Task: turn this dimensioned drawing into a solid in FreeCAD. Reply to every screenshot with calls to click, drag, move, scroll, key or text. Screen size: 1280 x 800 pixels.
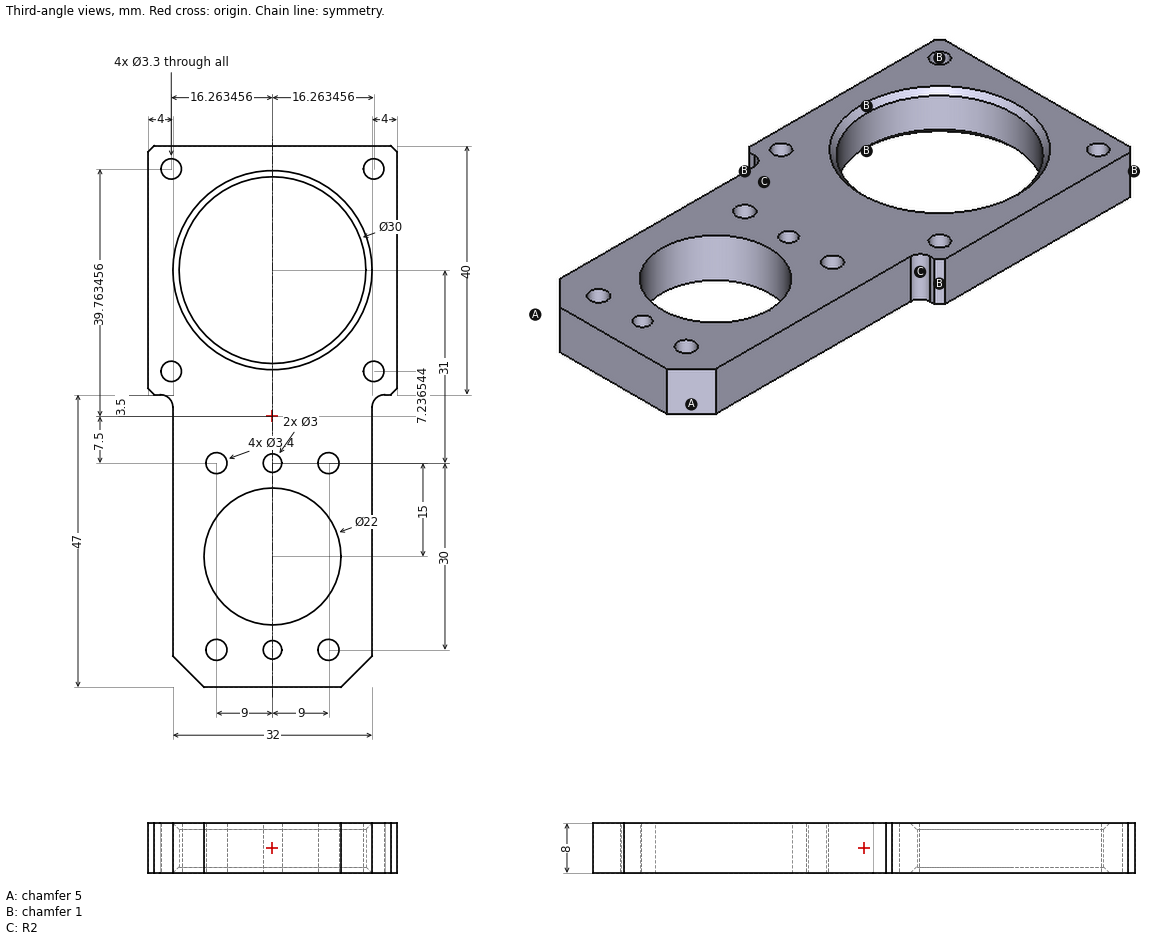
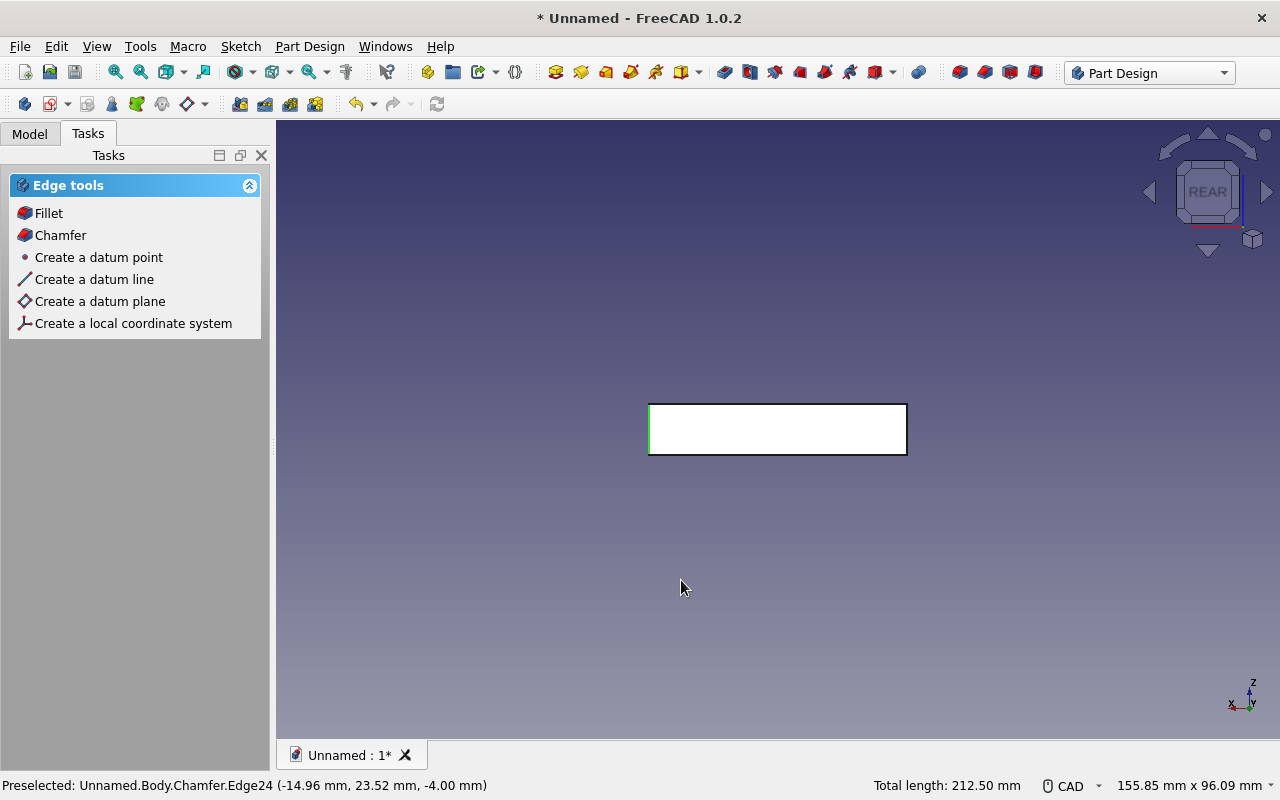
click(907, 429, ctrl)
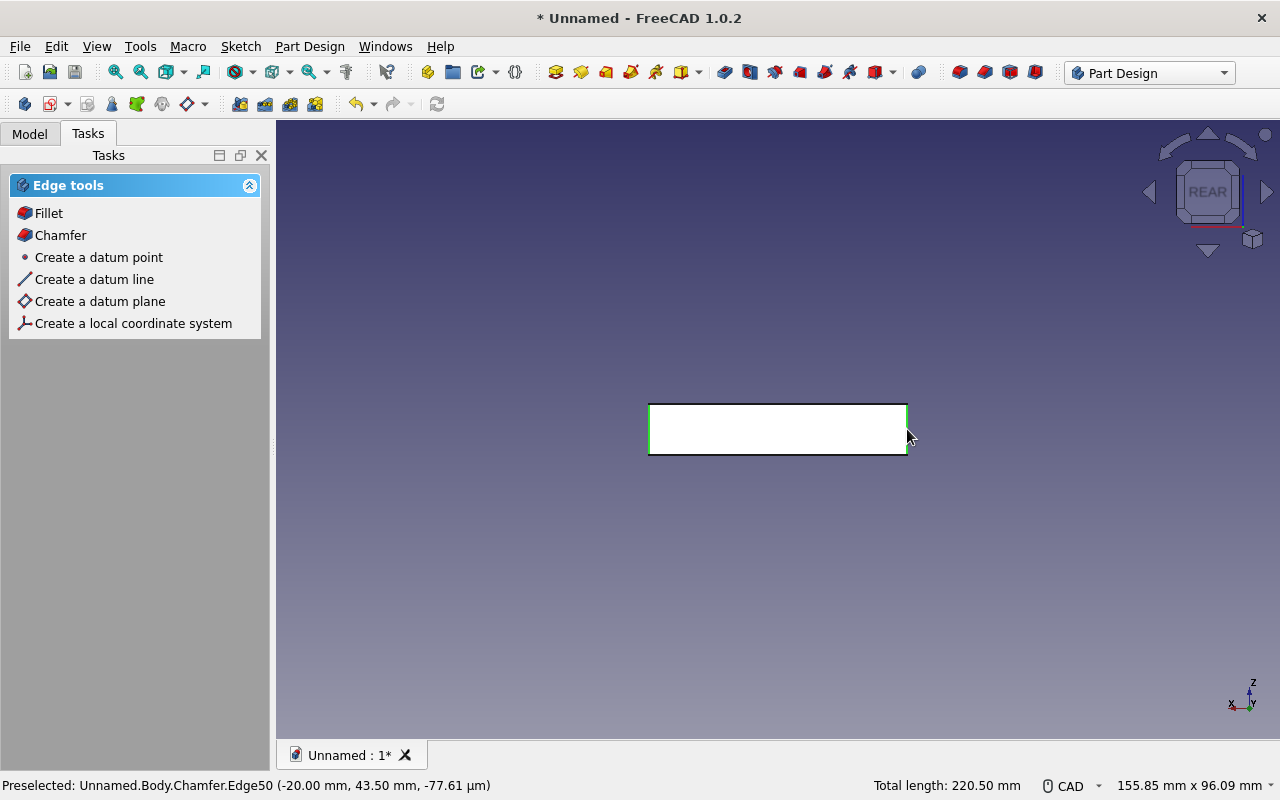
click(985, 72)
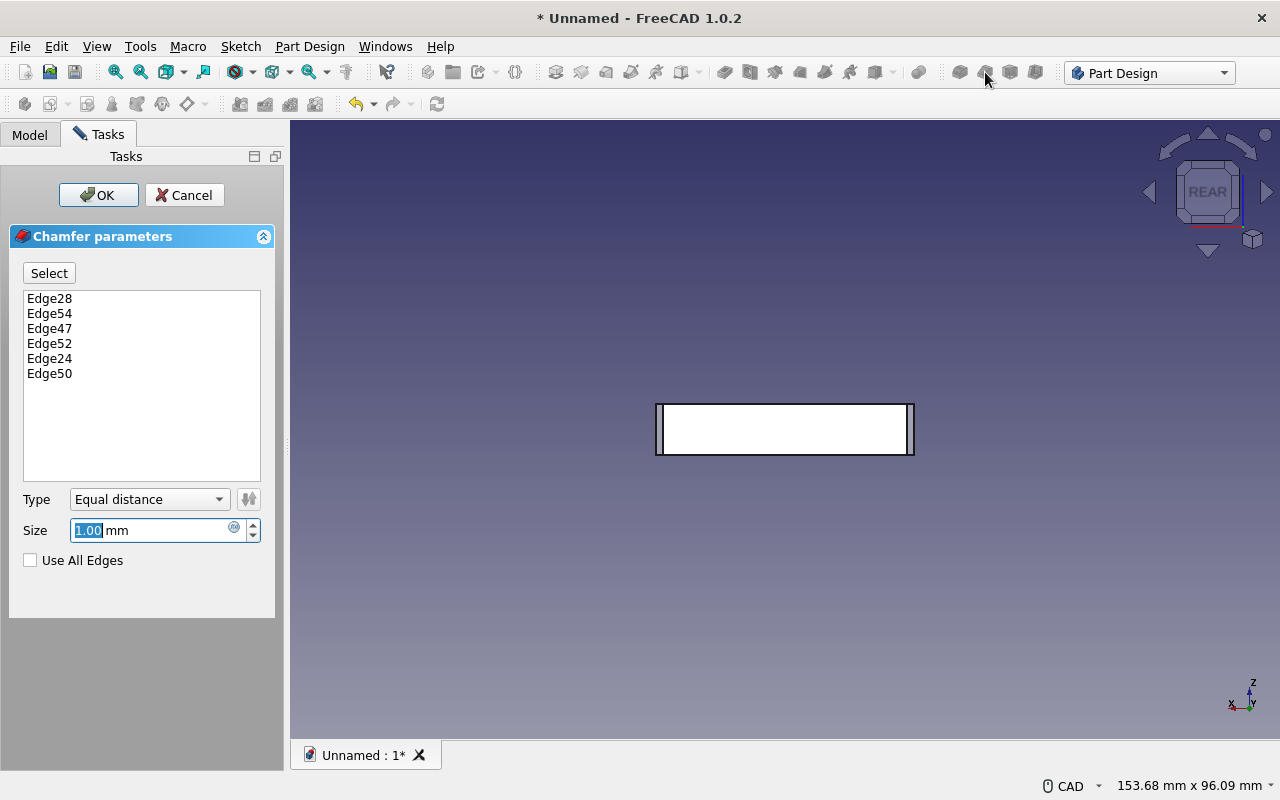
text(1)
key(Tab)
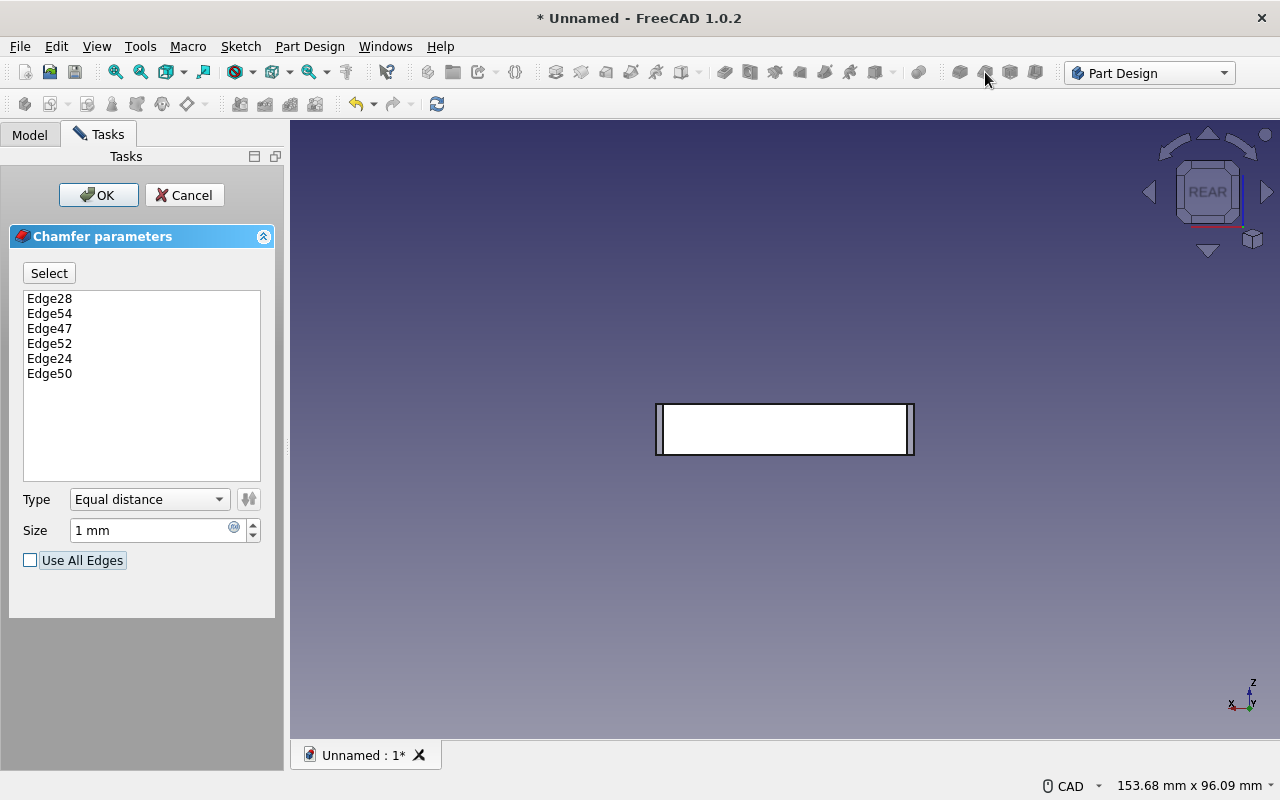
click(99, 195)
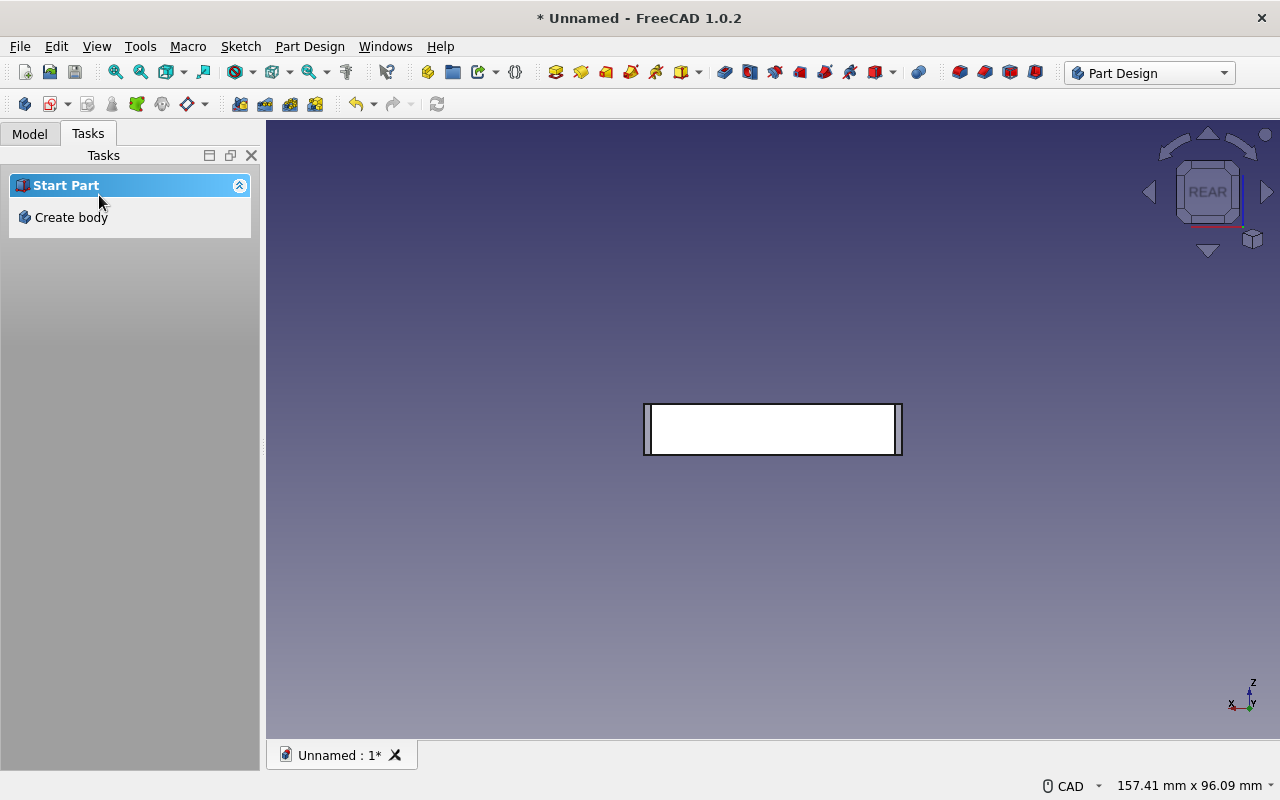
key(v)
key(f)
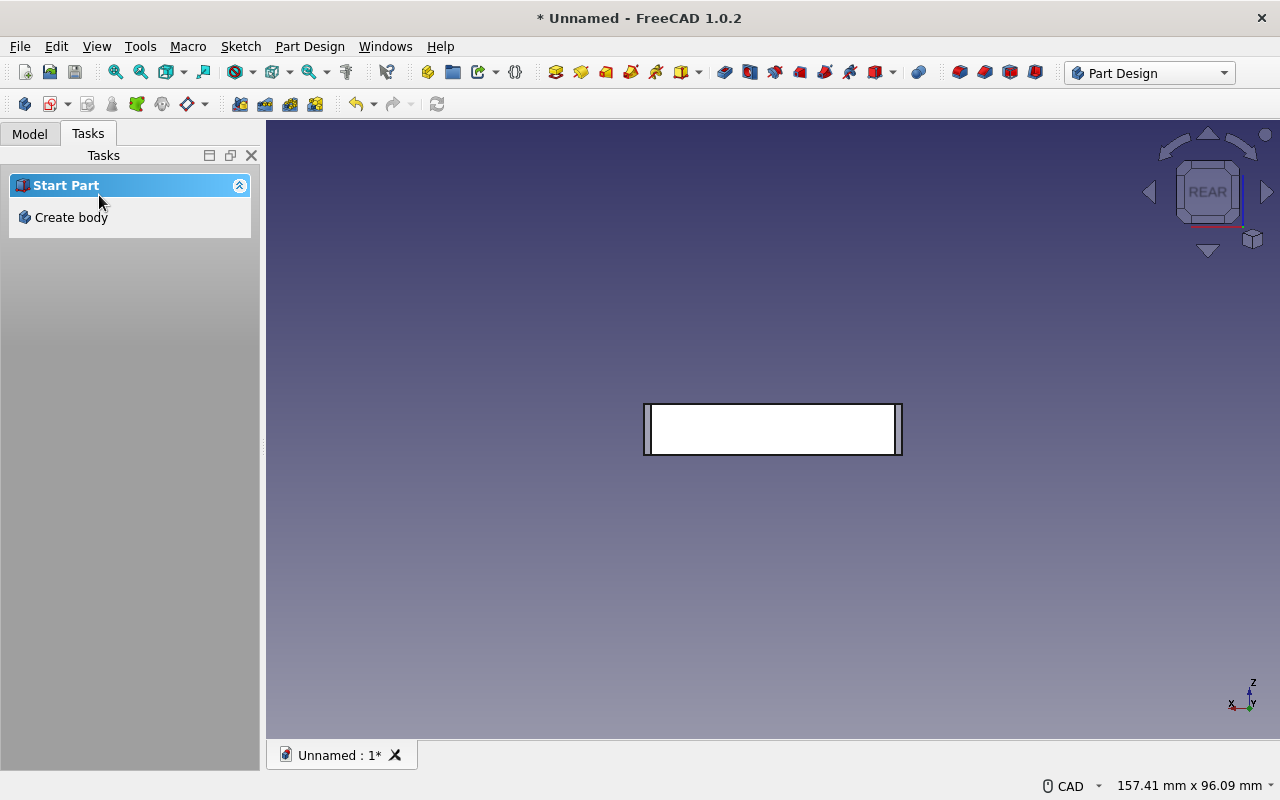
key(0)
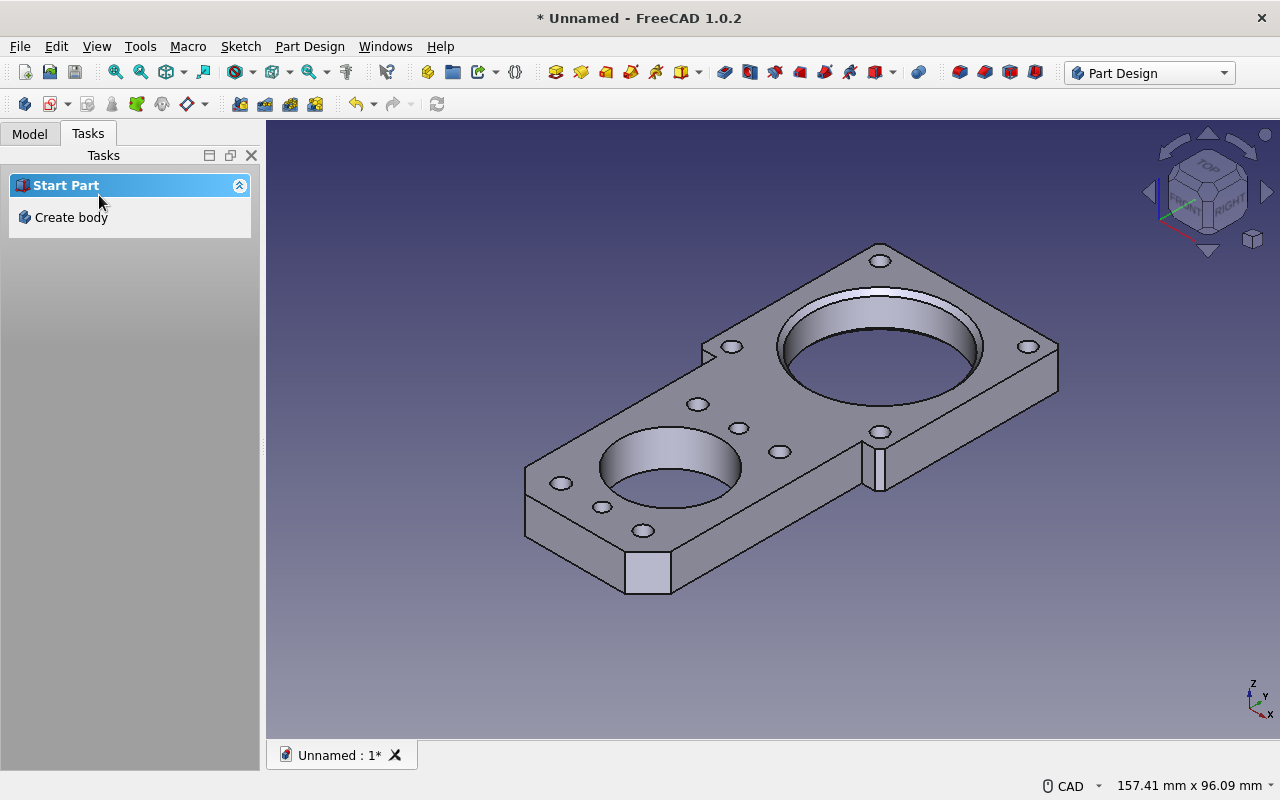
key(2)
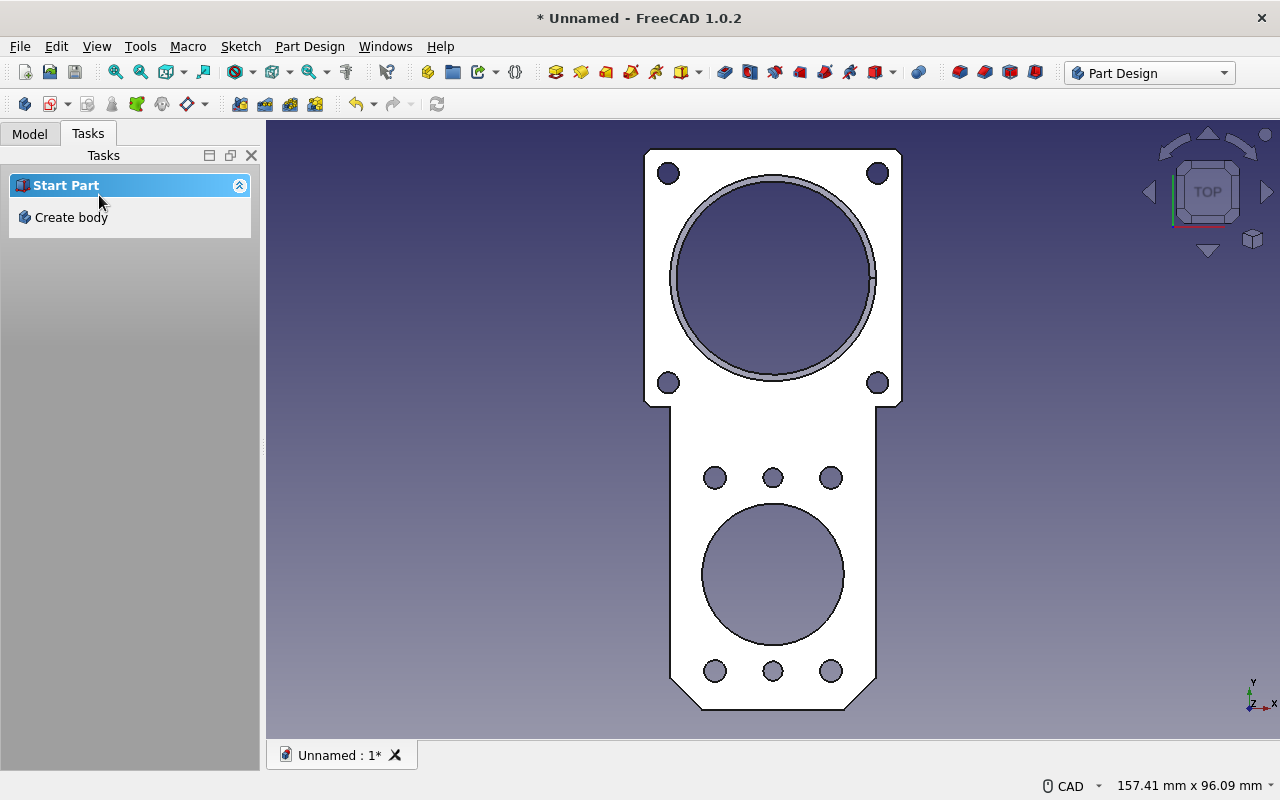
key(1)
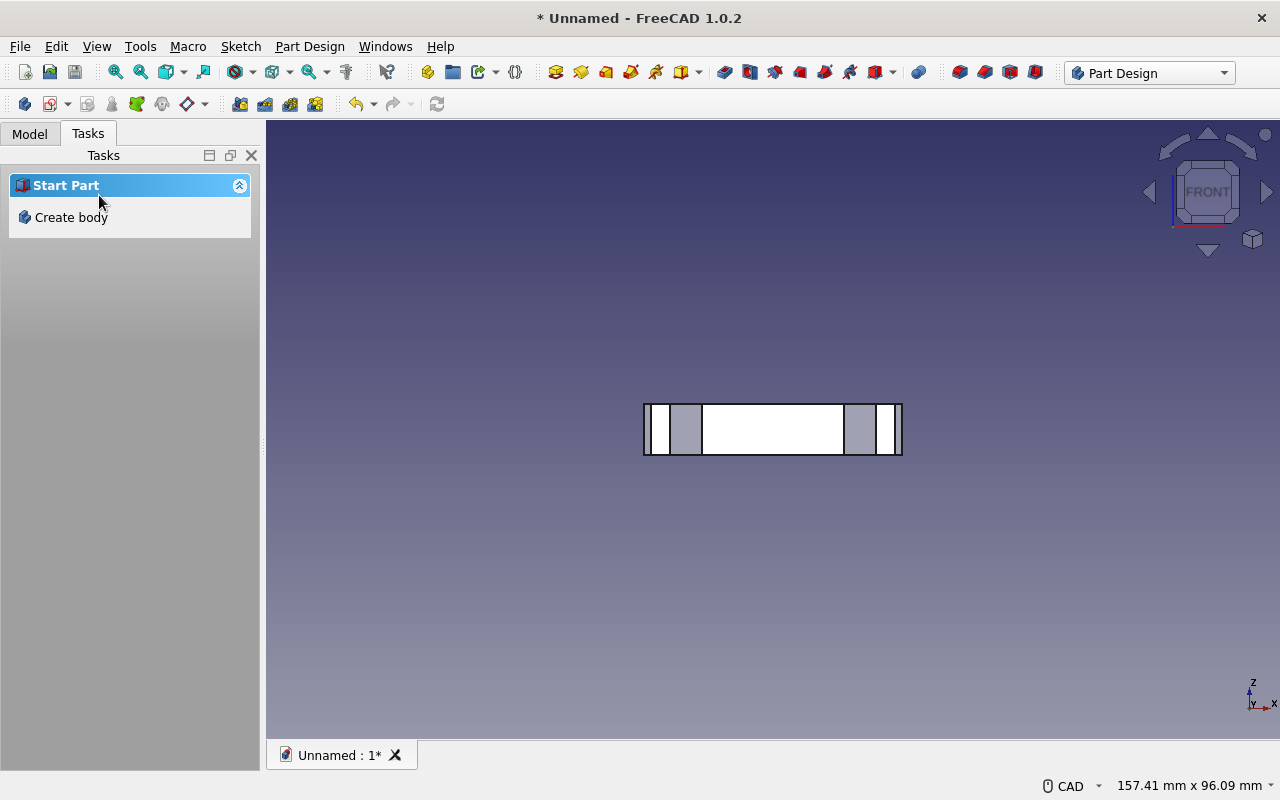
key(v)
key(f)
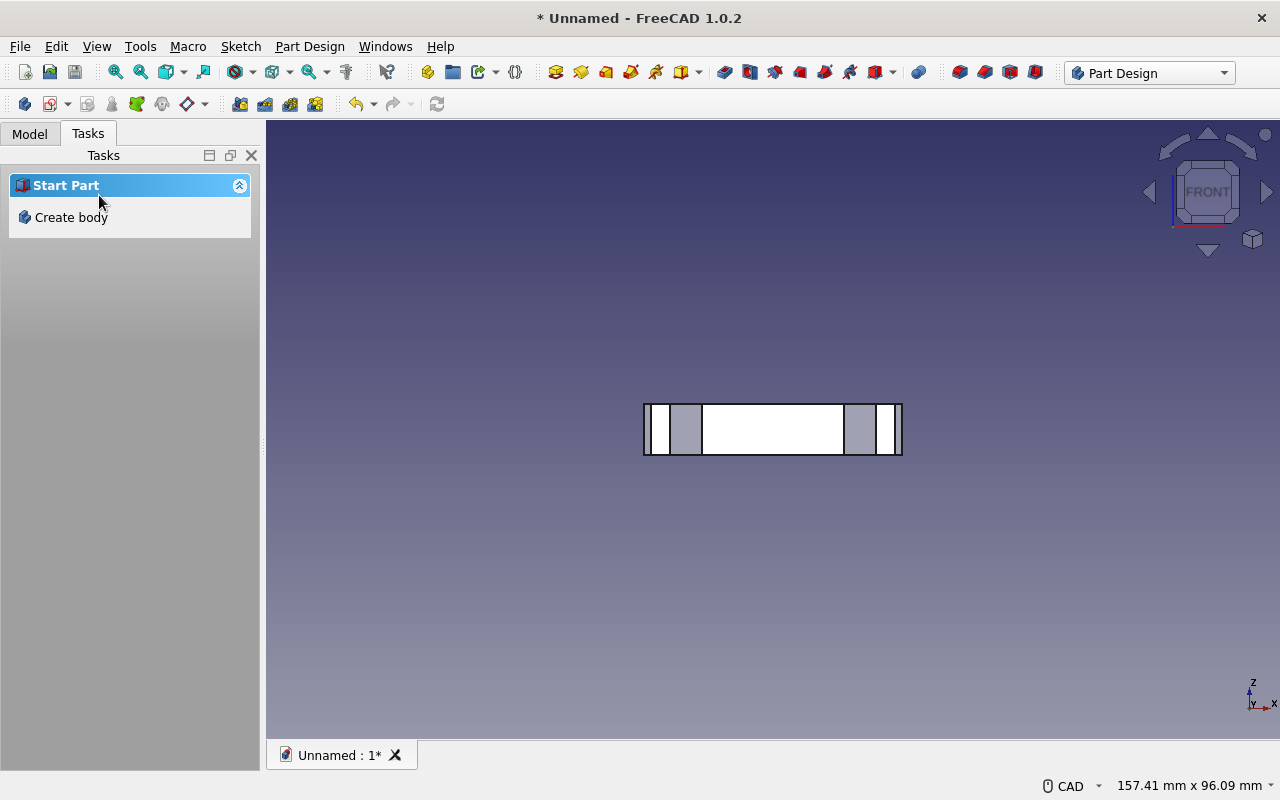
key(3)